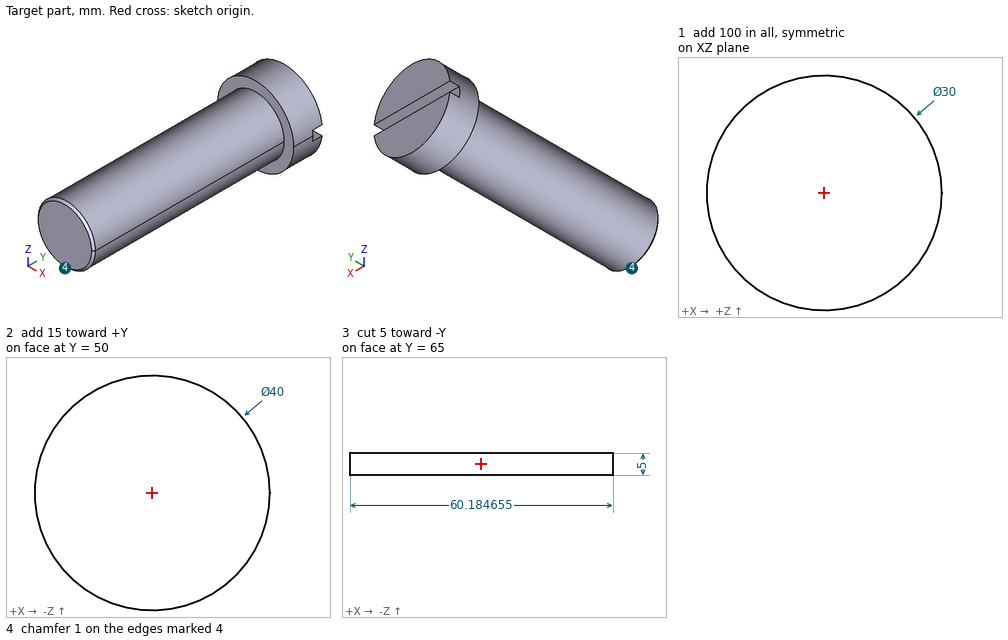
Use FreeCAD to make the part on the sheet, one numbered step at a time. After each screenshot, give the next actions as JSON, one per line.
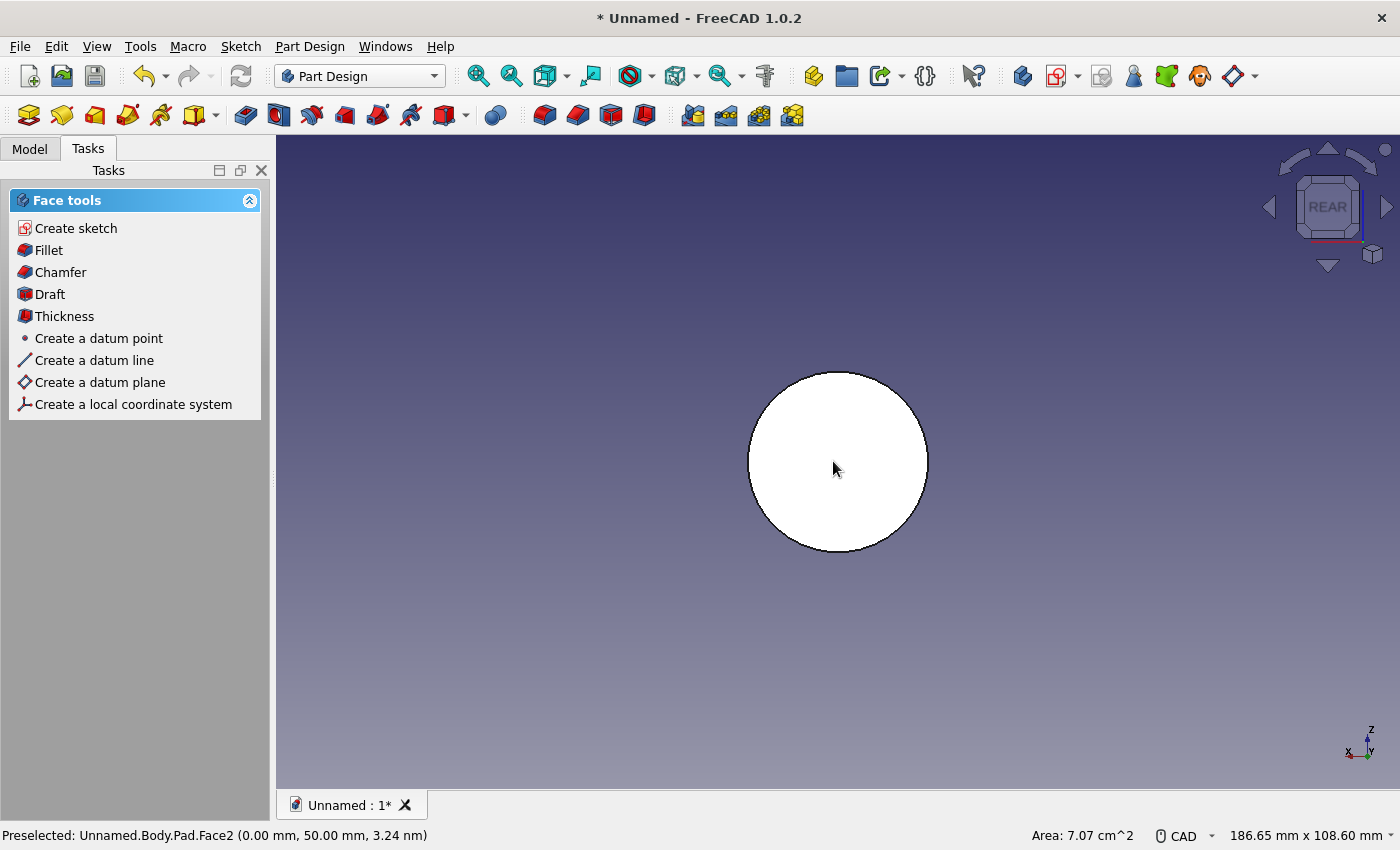
{"action": "left_click", "coordinate": [1056, 76]}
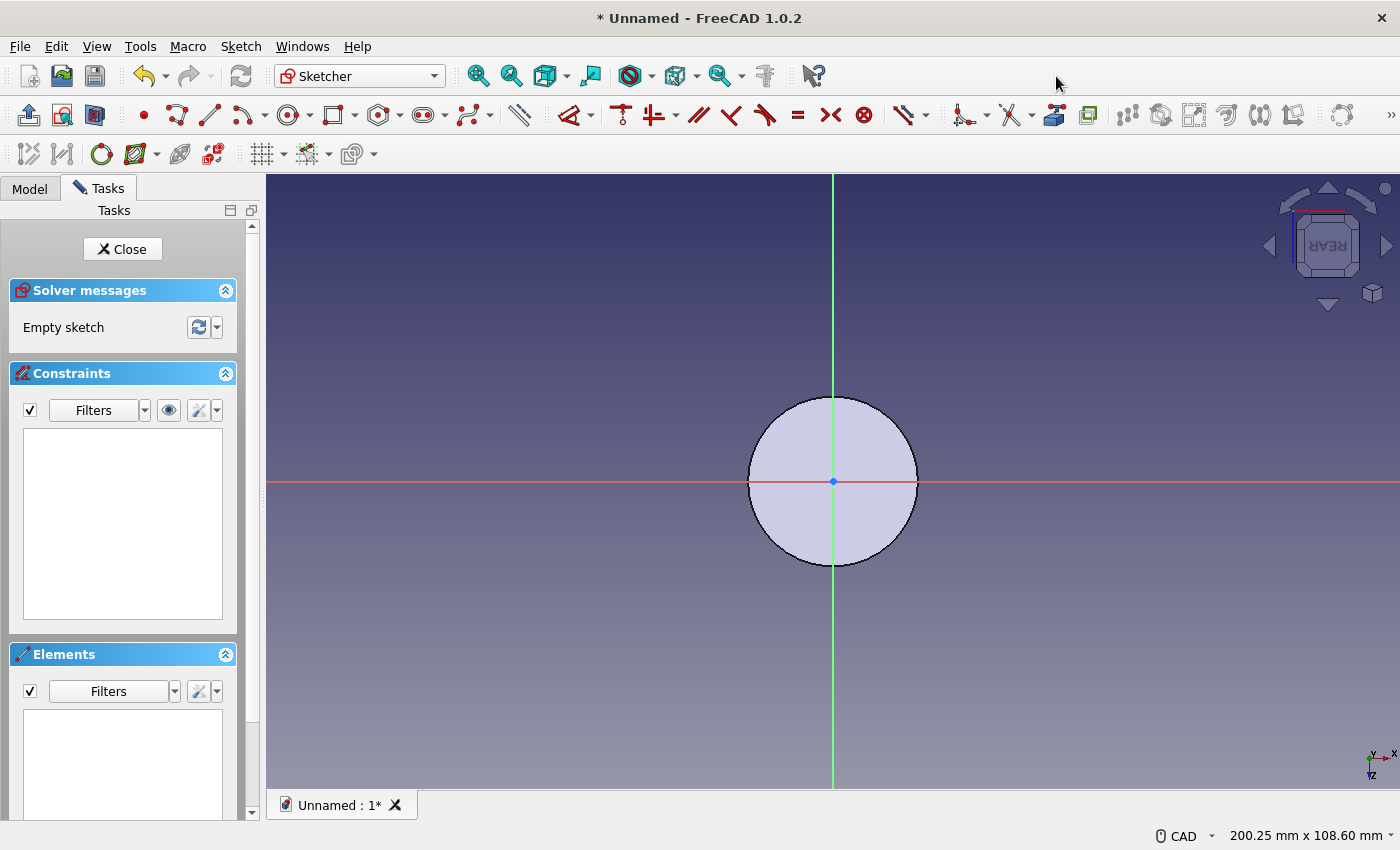
{"action": "scroll", "coordinate": [916, 481], "scroll_direction": "up", "scroll_amount": 3}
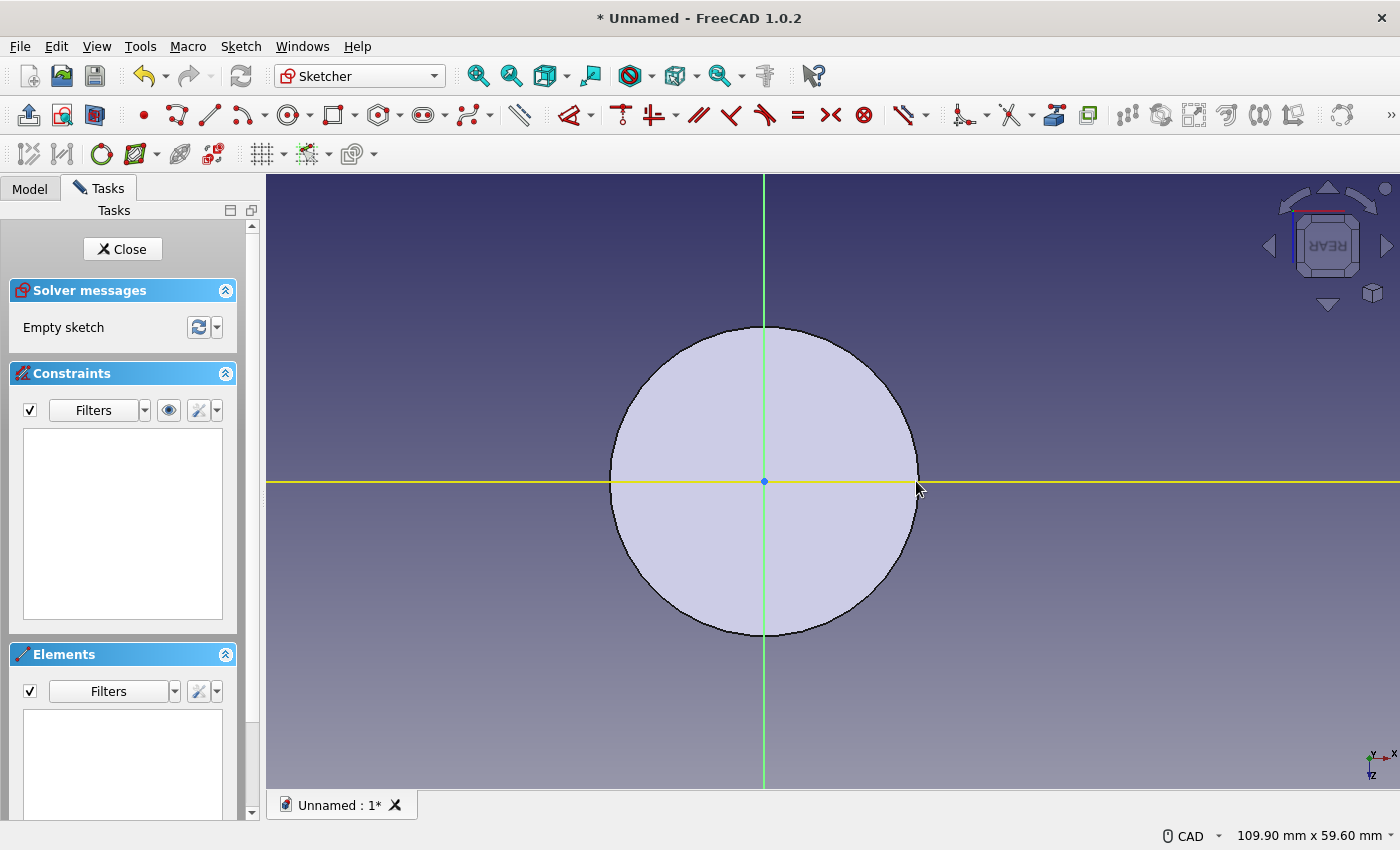
{"action": "left_click", "coordinate": [288, 116]}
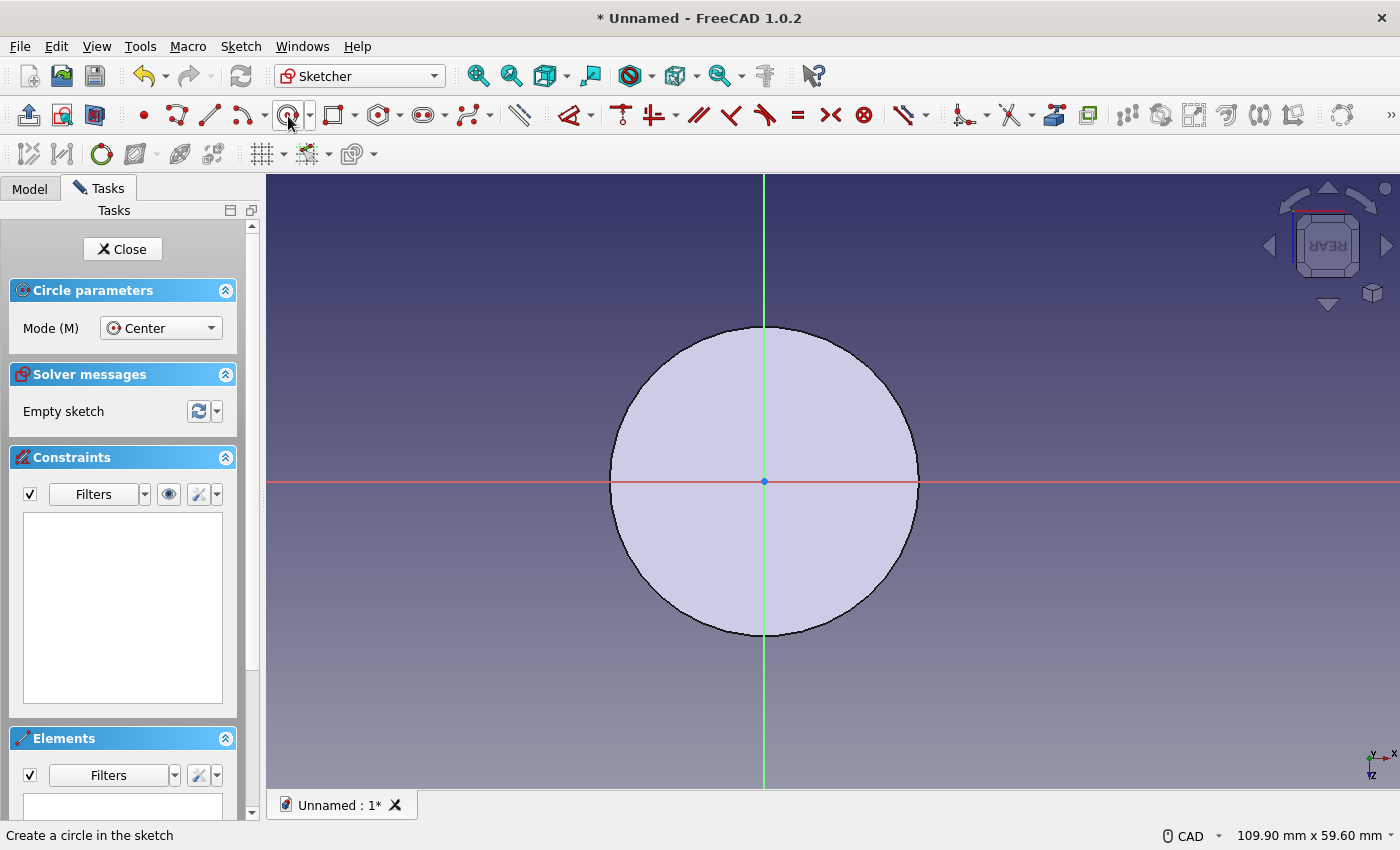
{"action": "left_click", "coordinate": [764, 481]}
{"action": "left_click", "coordinate": [910, 336]}
{"action": "key", "text": "Escape"}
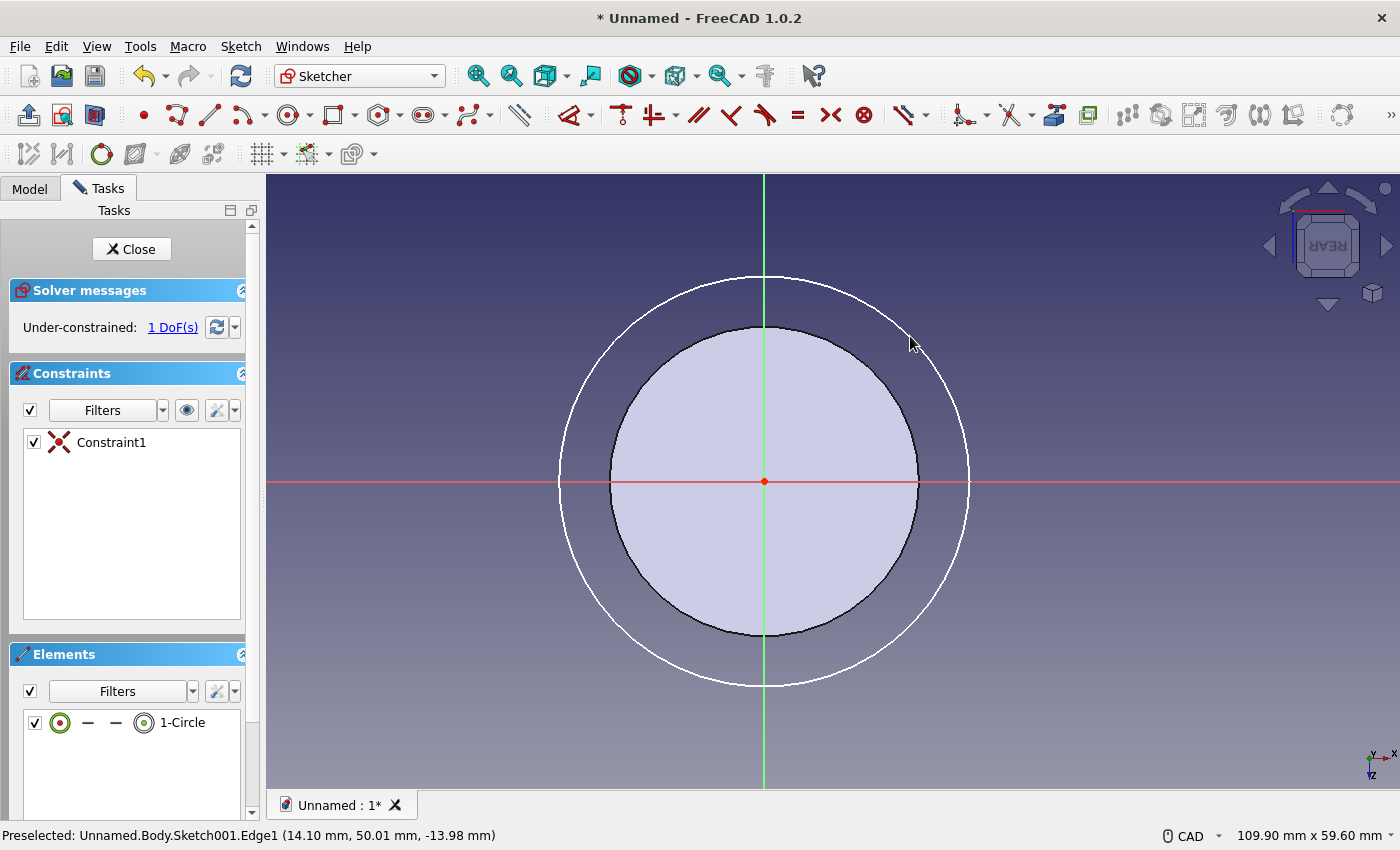
{"action": "left_click", "coordinate": [568, 116]}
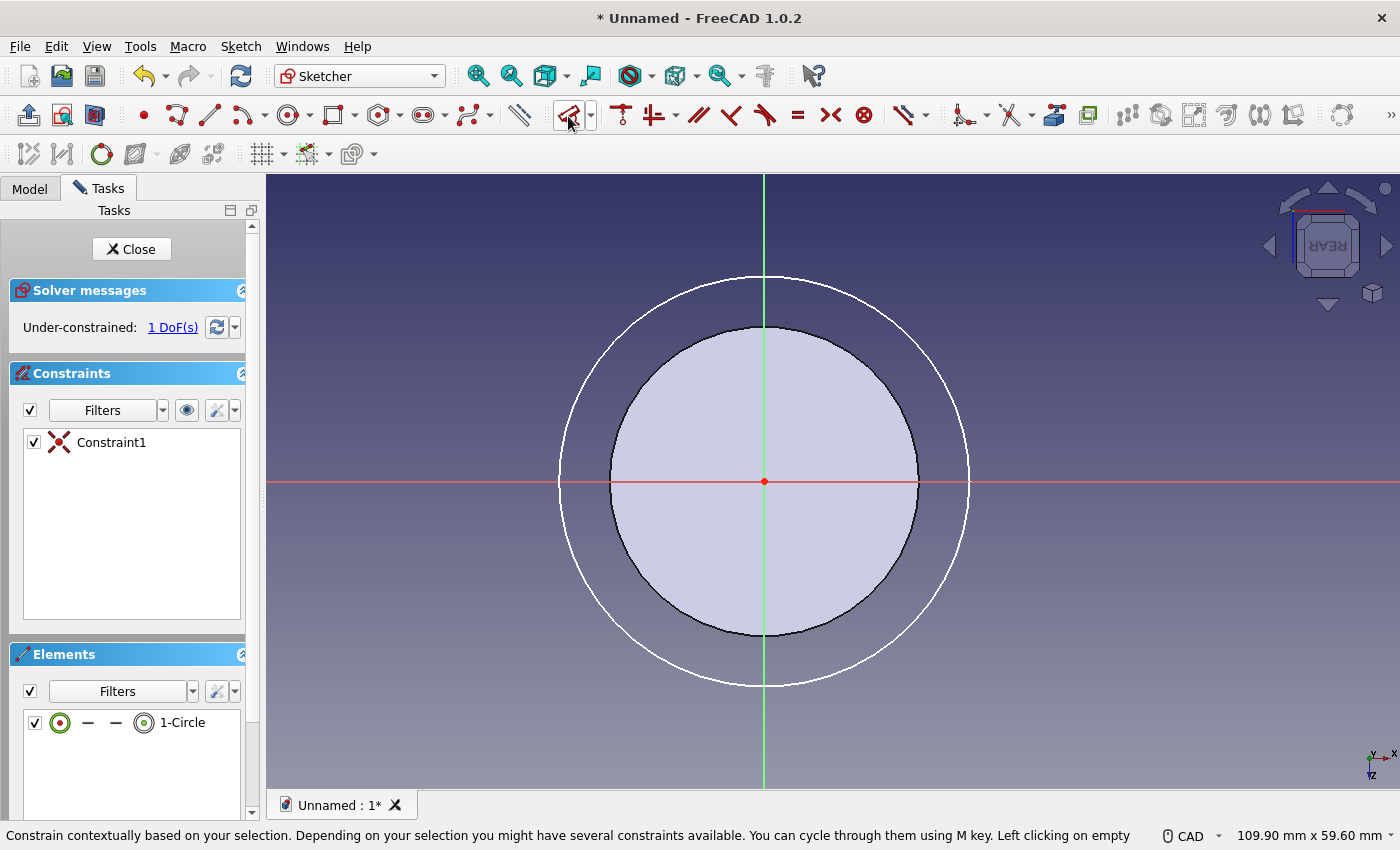
{"action": "left_click", "coordinate": [909, 336]}
{"action": "left_click", "coordinate": [932, 313]}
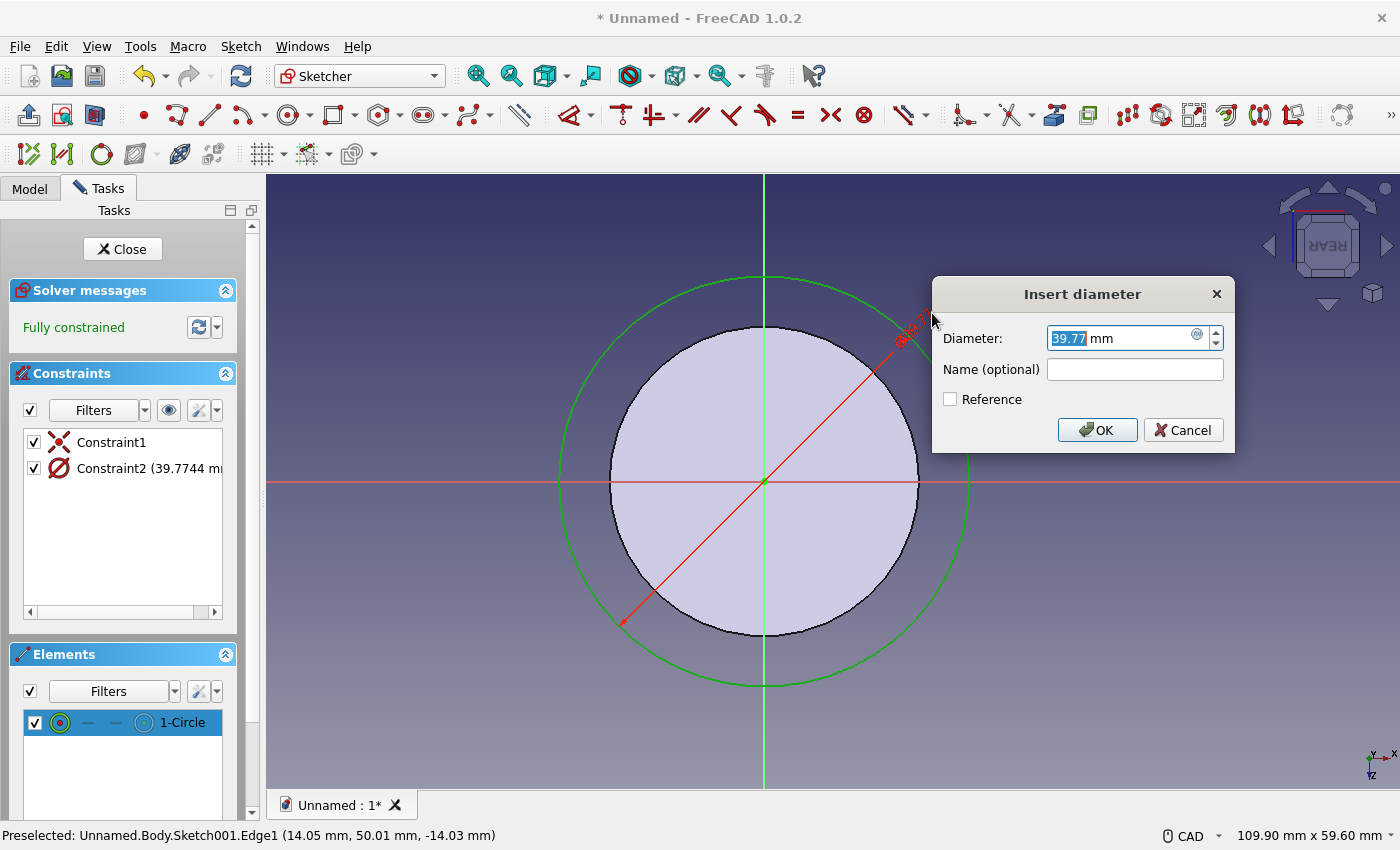
{"action": "type", "text": "40"}
{"action": "key", "text": "Return"}
{"action": "key", "text": "Escape"}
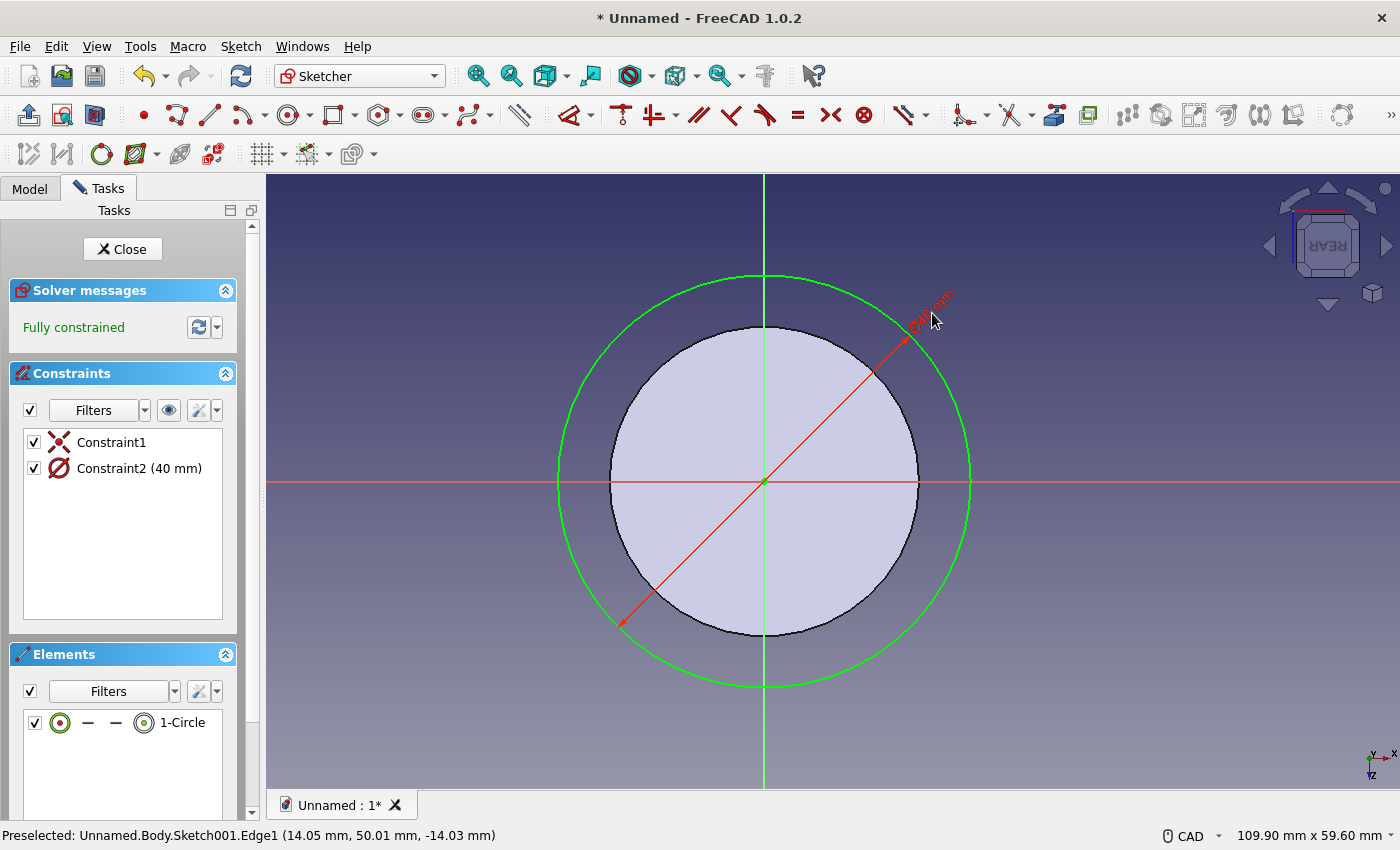
{"action": "left_click", "coordinate": [123, 249]}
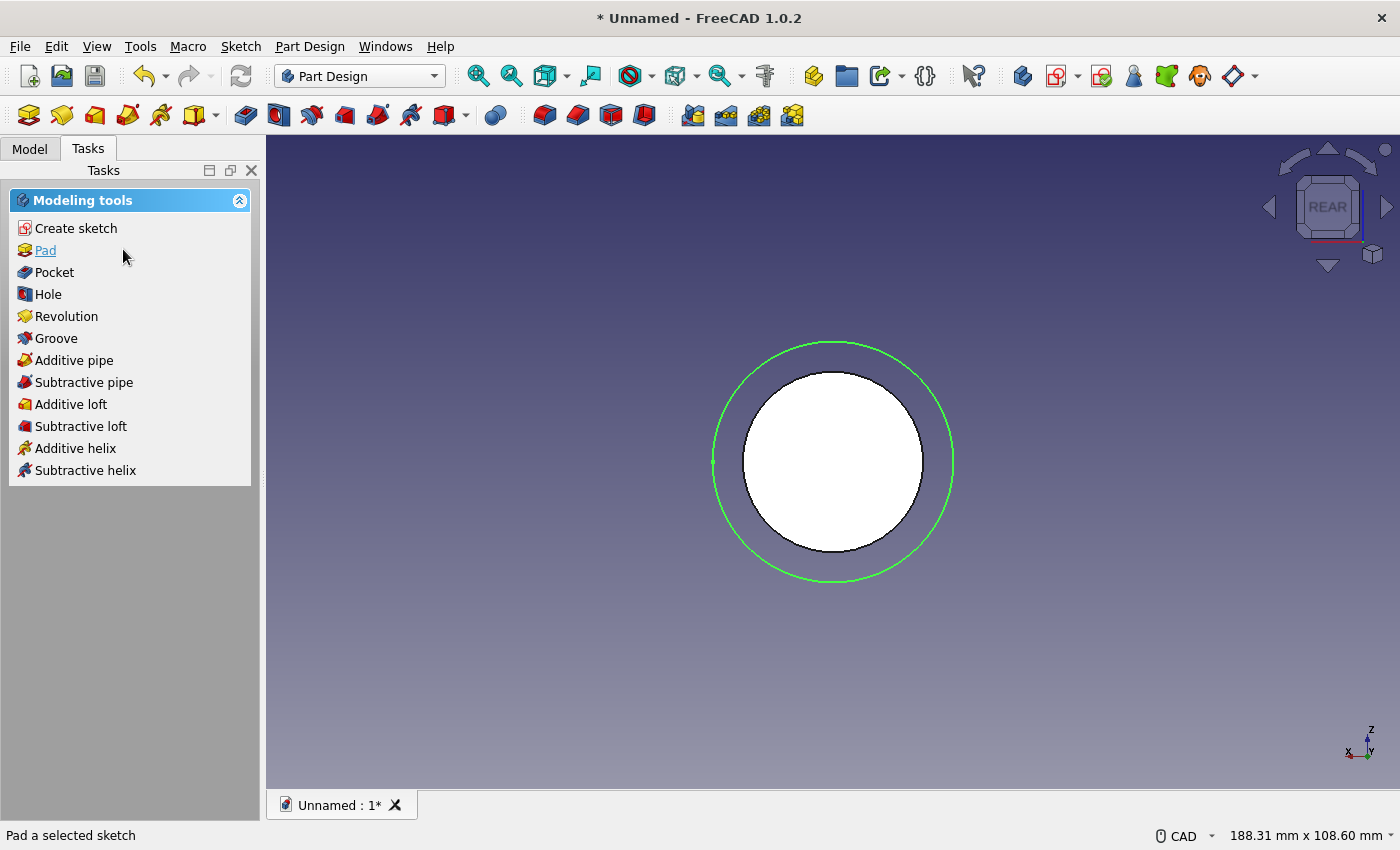
{"action": "left_click", "coordinate": [29, 116]}